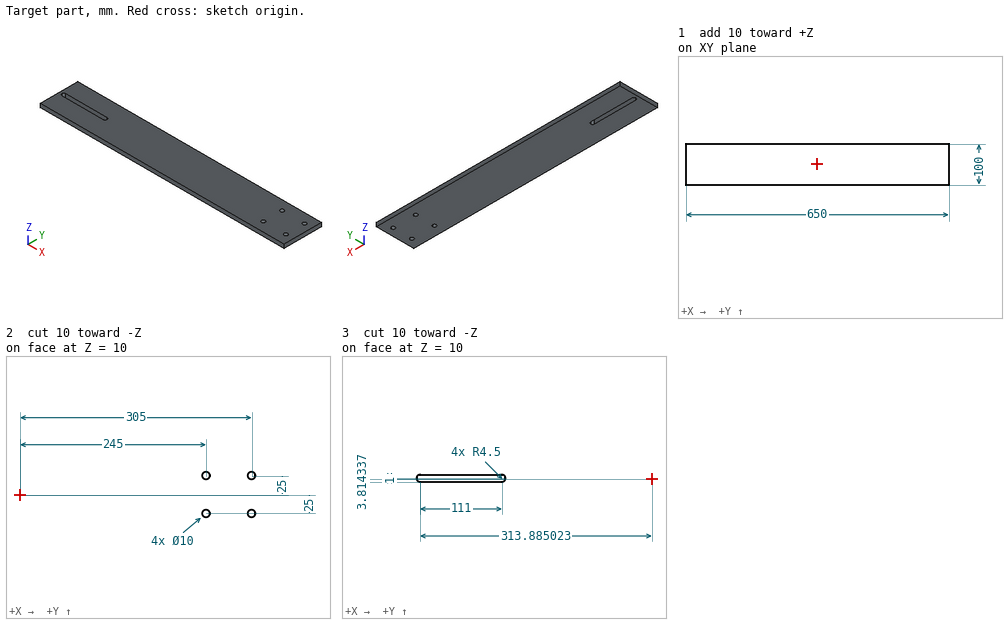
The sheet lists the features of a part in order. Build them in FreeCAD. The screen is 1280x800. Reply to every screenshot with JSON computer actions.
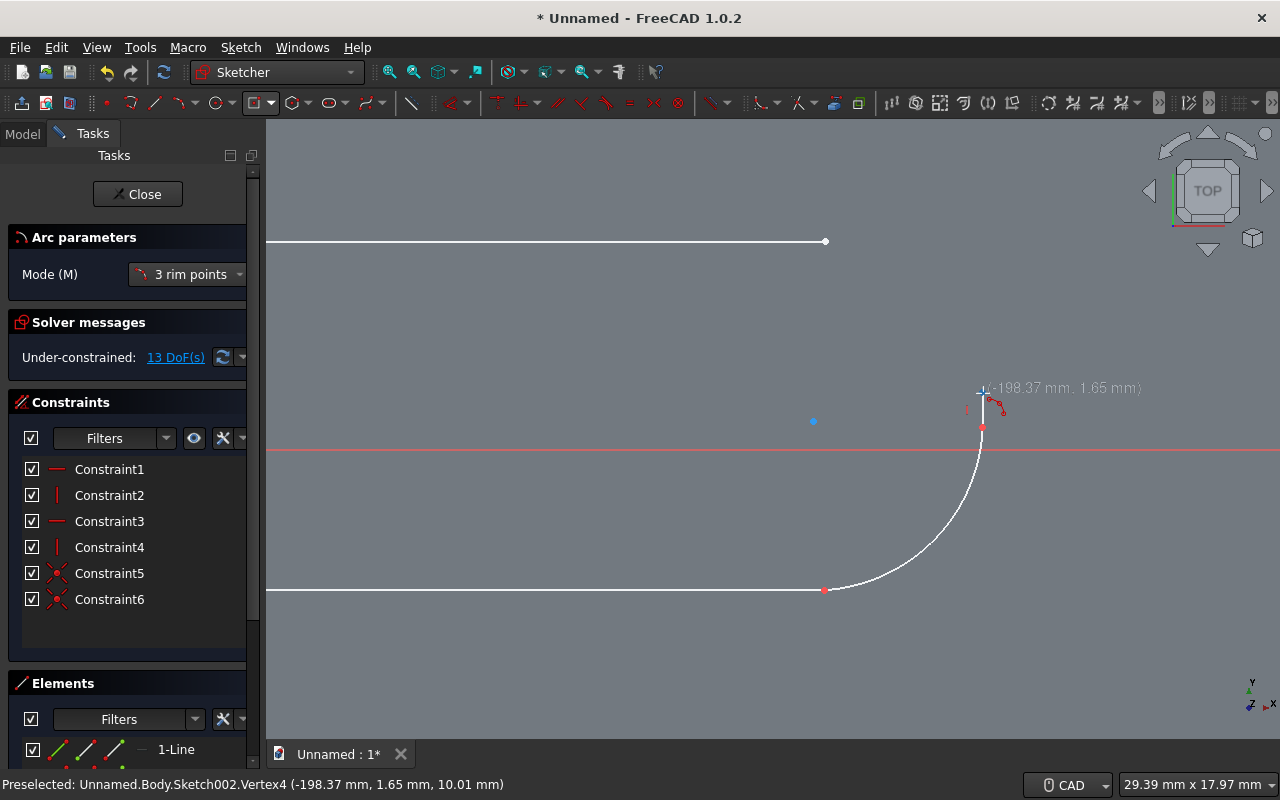
{"action": "scroll", "coordinate": [985, 432], "scroll_direction": "down", "scroll_amount": 10}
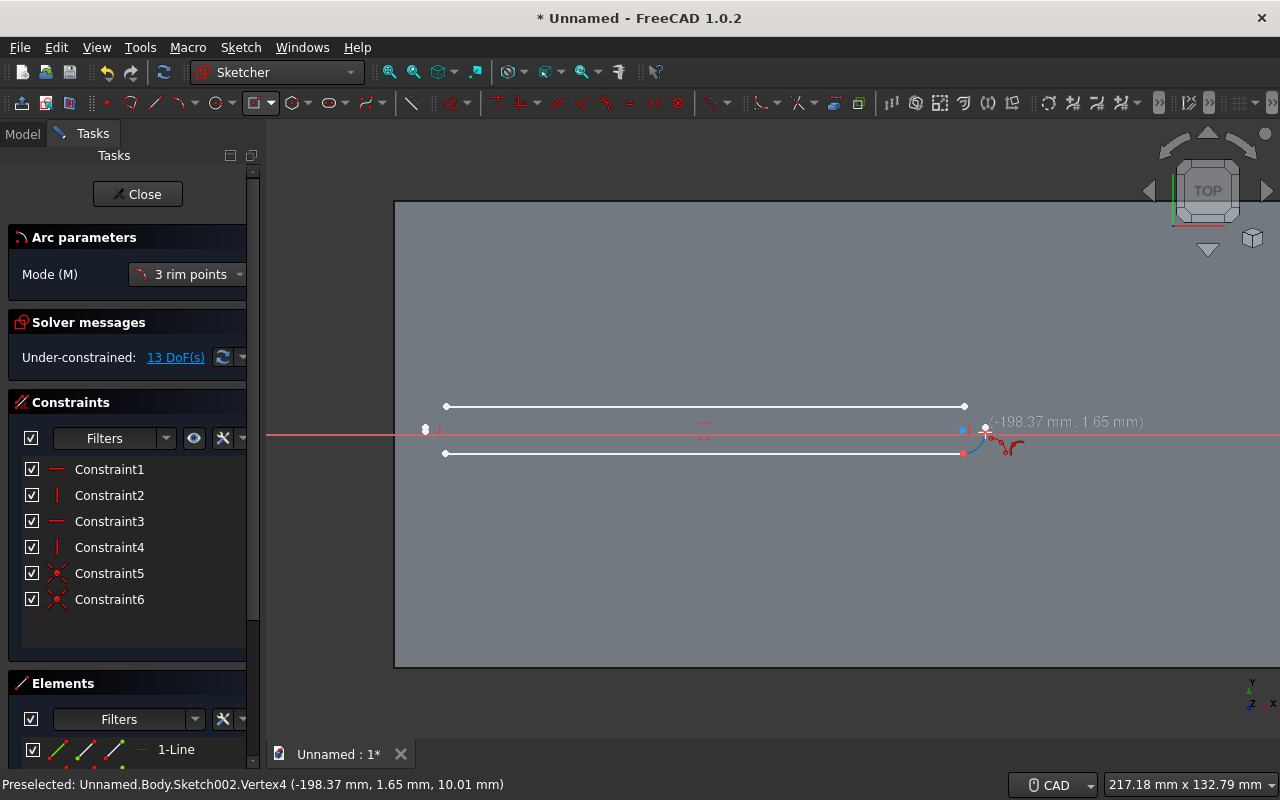
{"action": "left_click", "coordinate": [964, 407]}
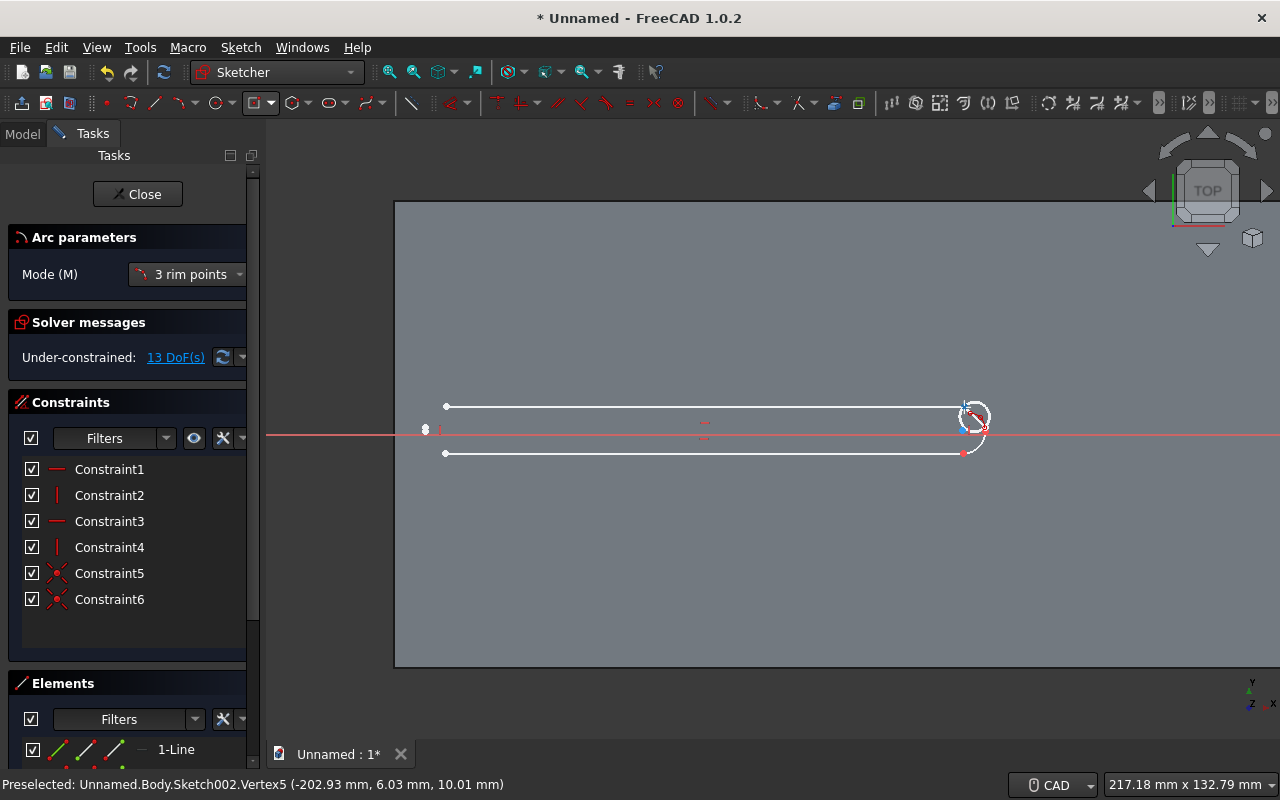
{"action": "scroll", "coordinate": [979, 412], "scroll_direction": "up", "scroll_amount": 5}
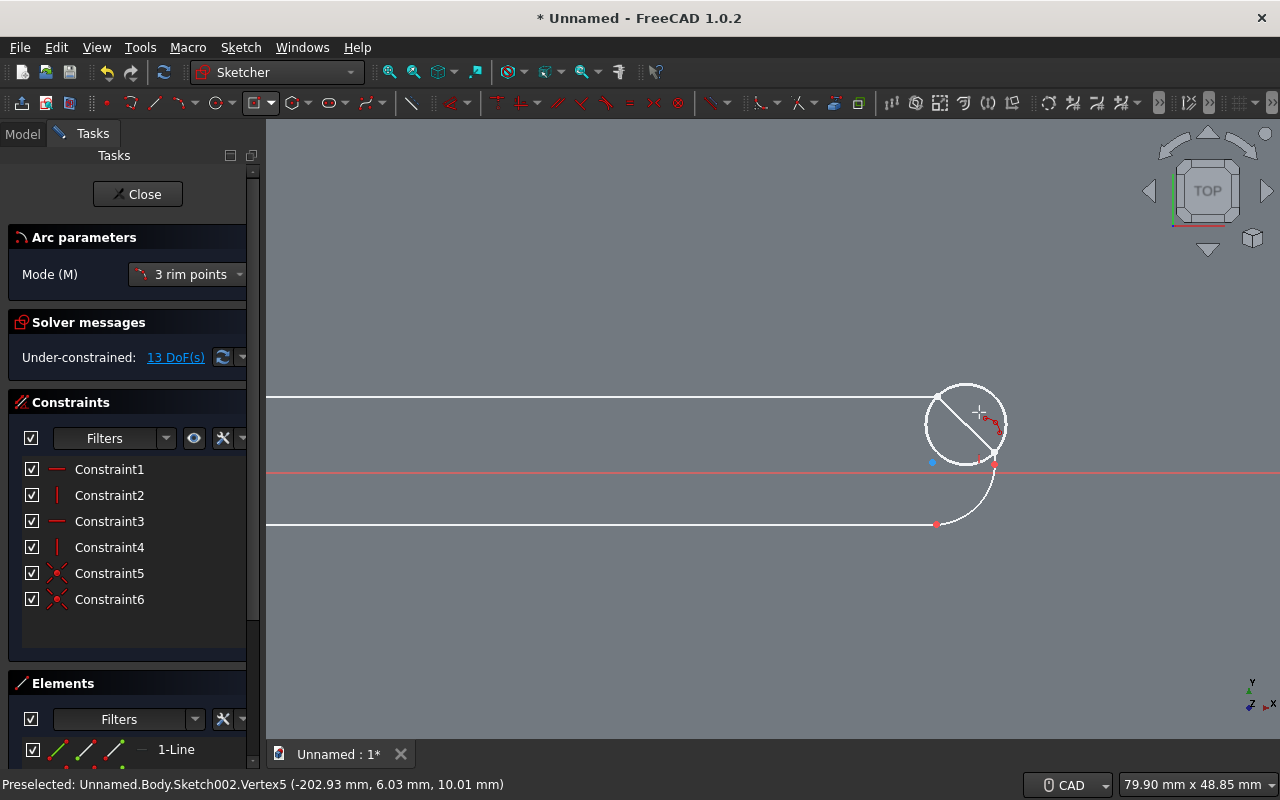
{"action": "left_click", "coordinate": [978, 411]}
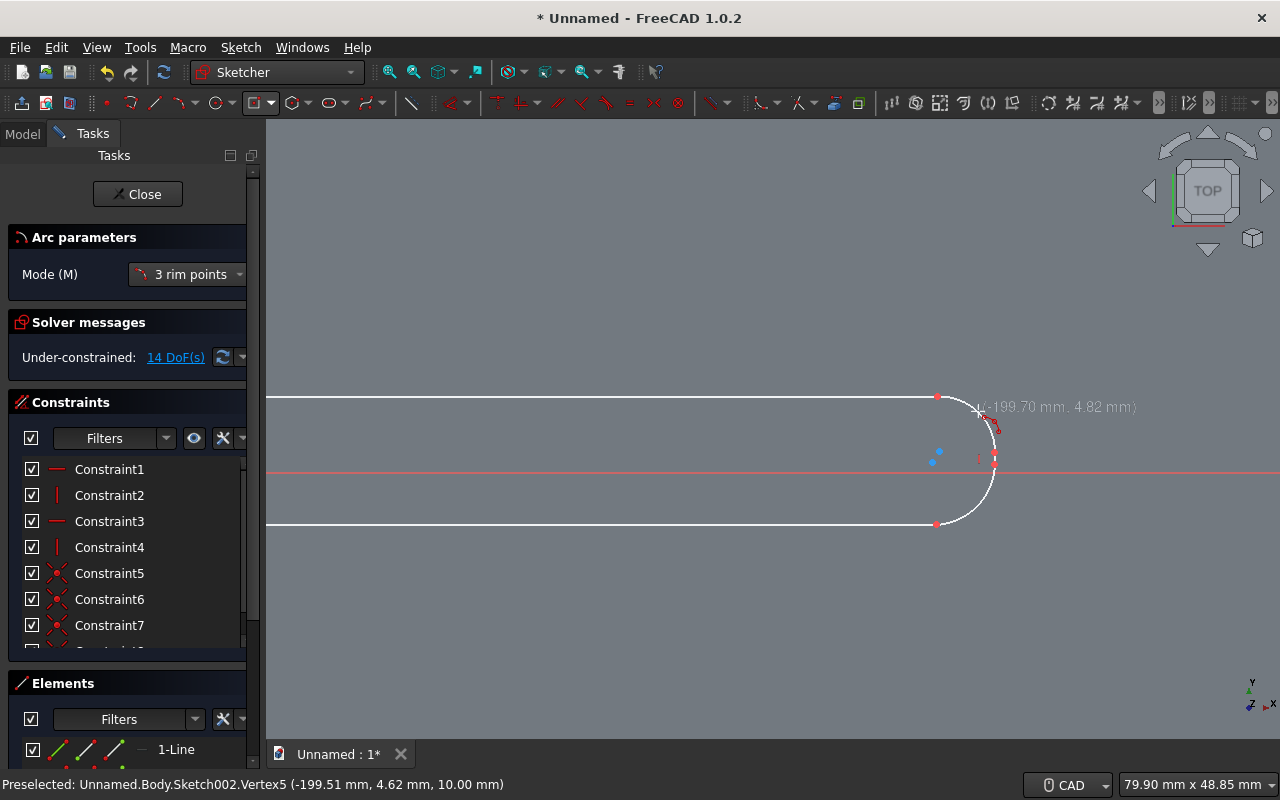
{"action": "scroll", "coordinate": [979, 412], "scroll_direction": "down", "scroll_amount": 5}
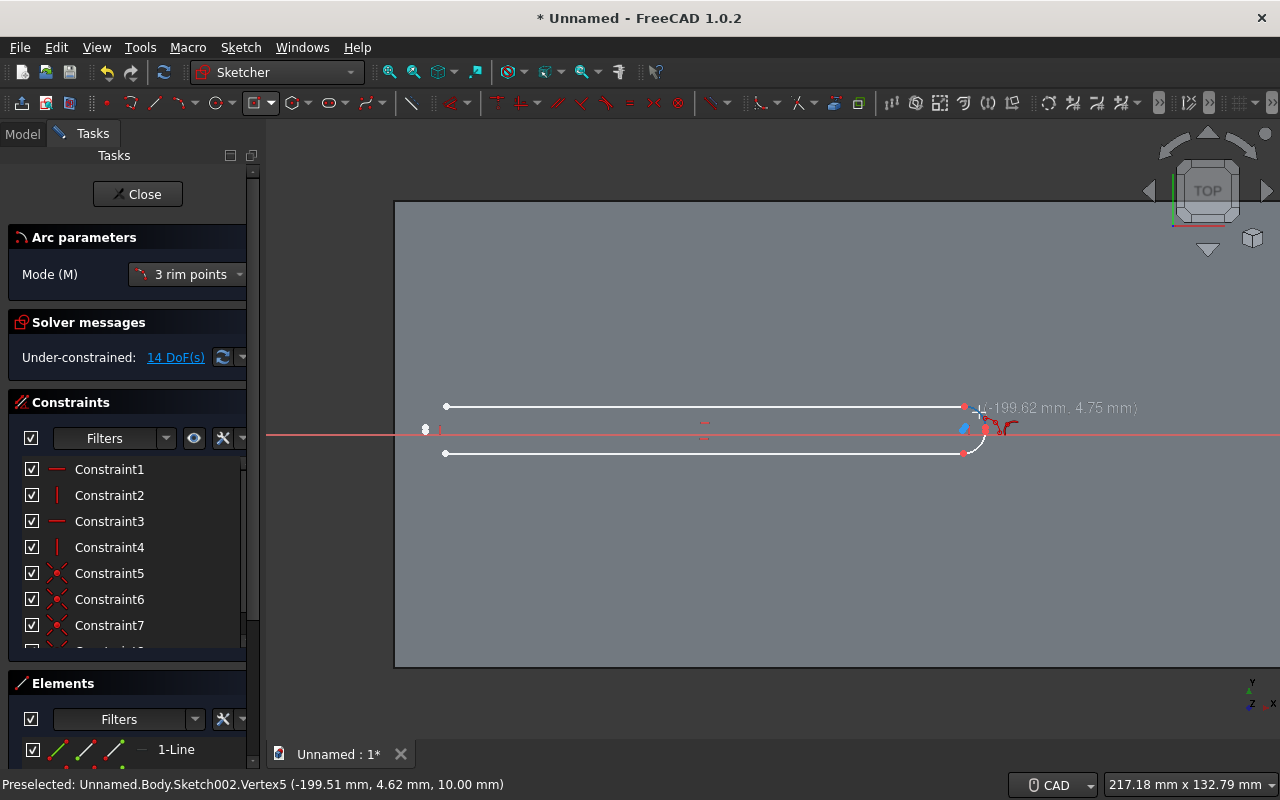
{"action": "left_click", "coordinate": [446, 407]}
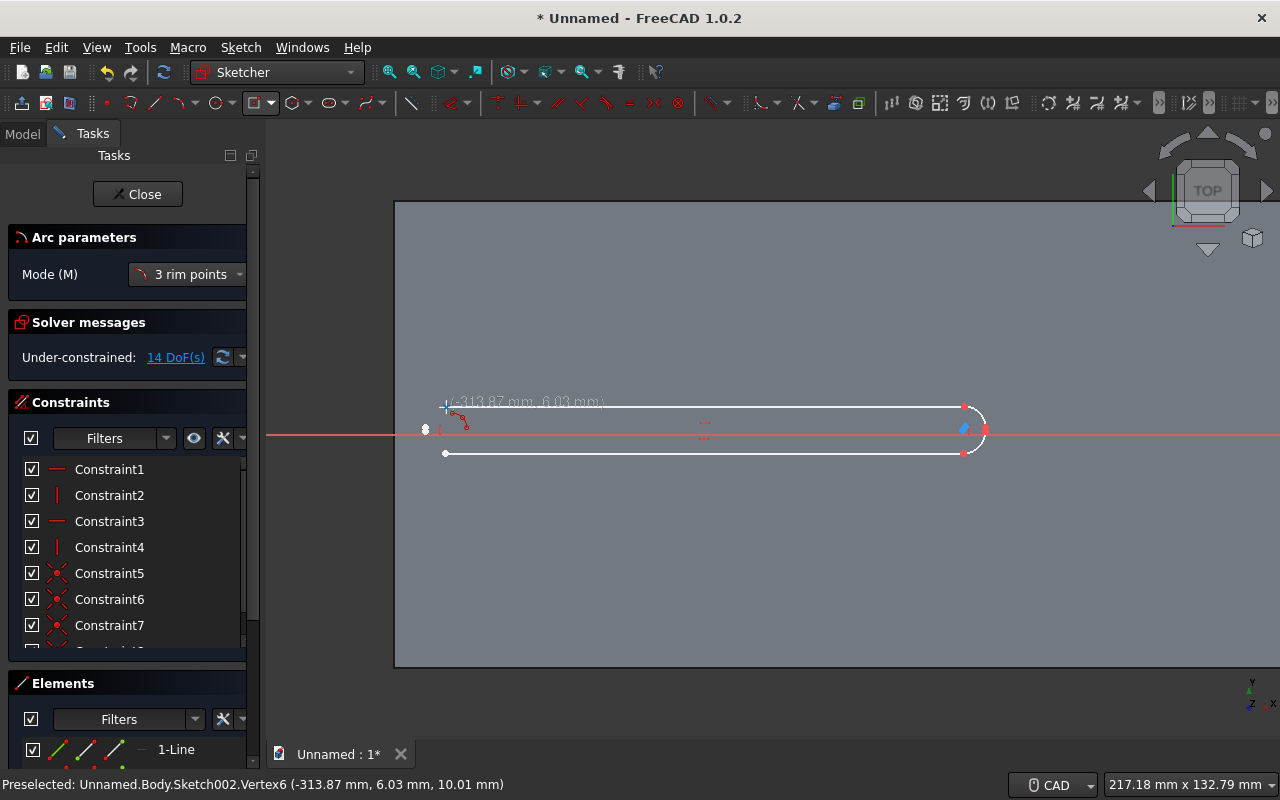
{"action": "scroll", "coordinate": [425, 427], "scroll_direction": "up", "scroll_amount": 10}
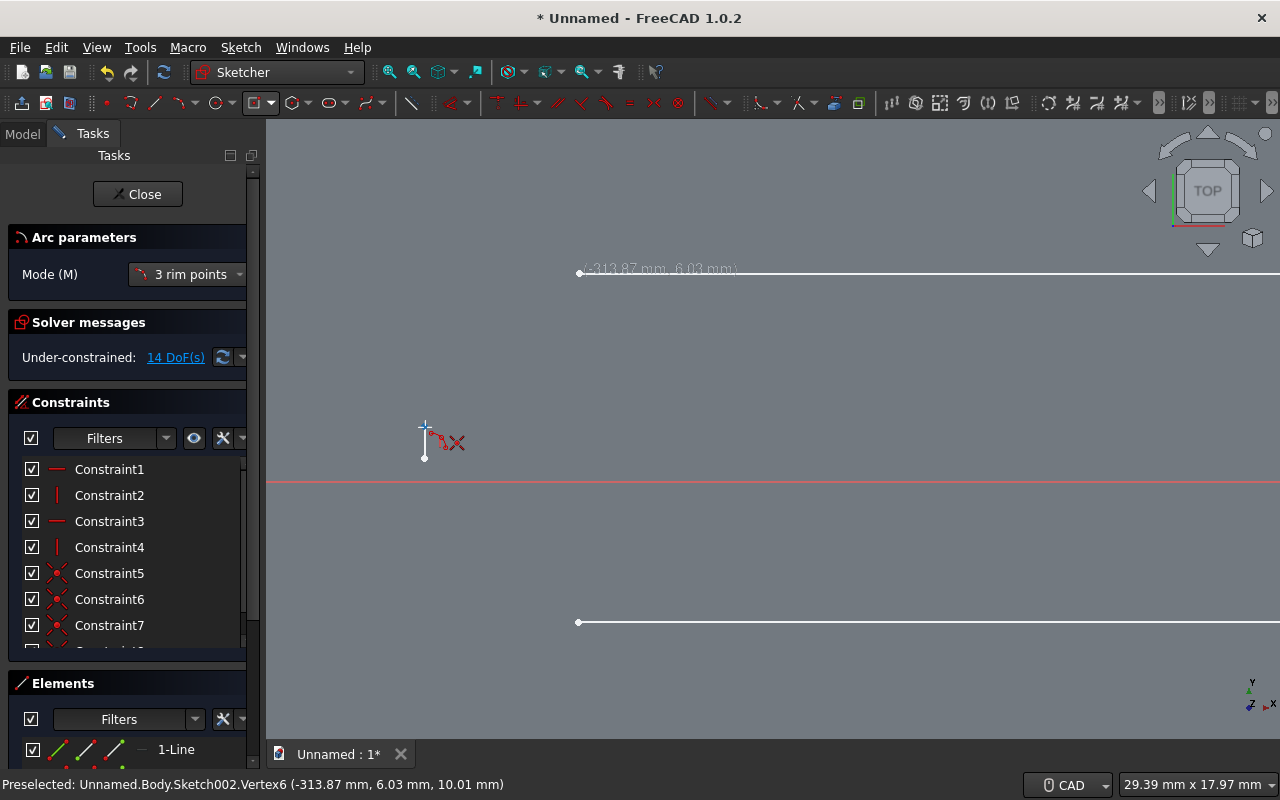
{"action": "left_click", "coordinate": [425, 427]}
{"action": "left_click", "coordinate": [469, 314]}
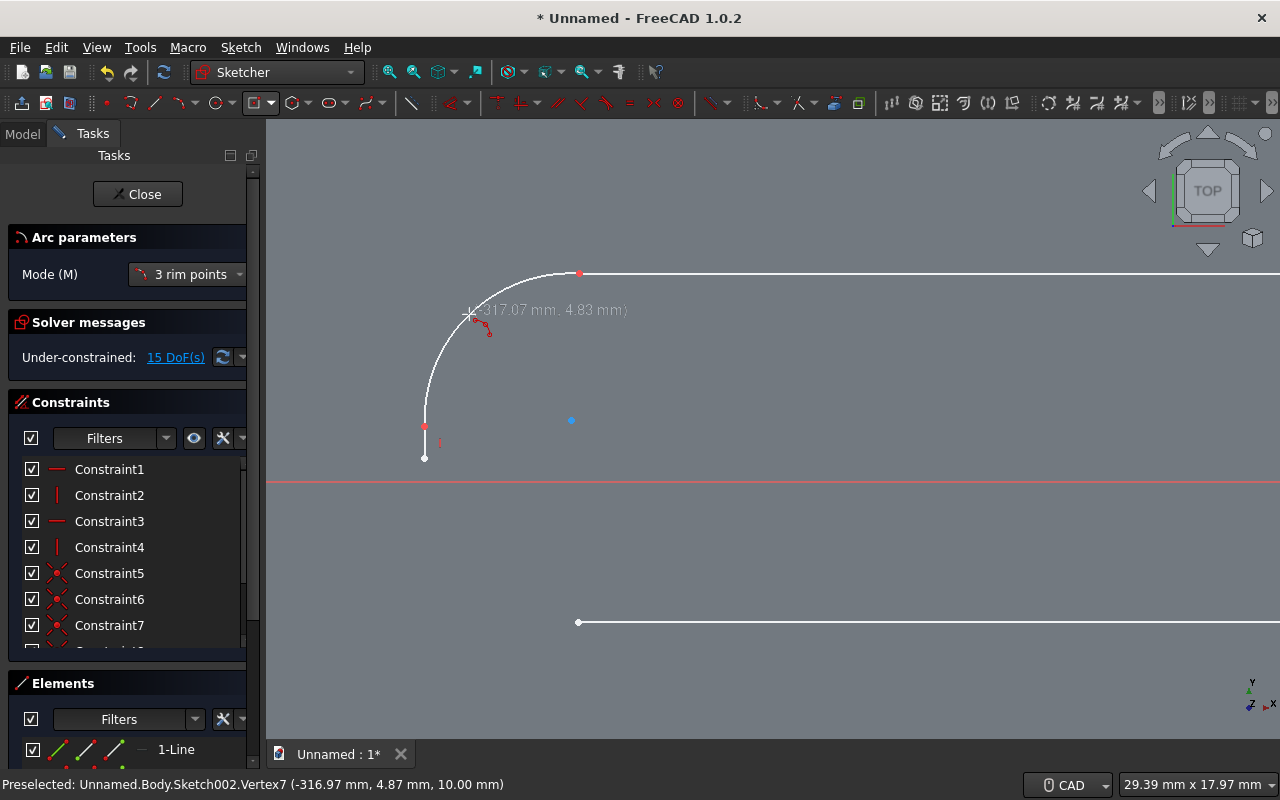
{"action": "left_click", "coordinate": [425, 459]}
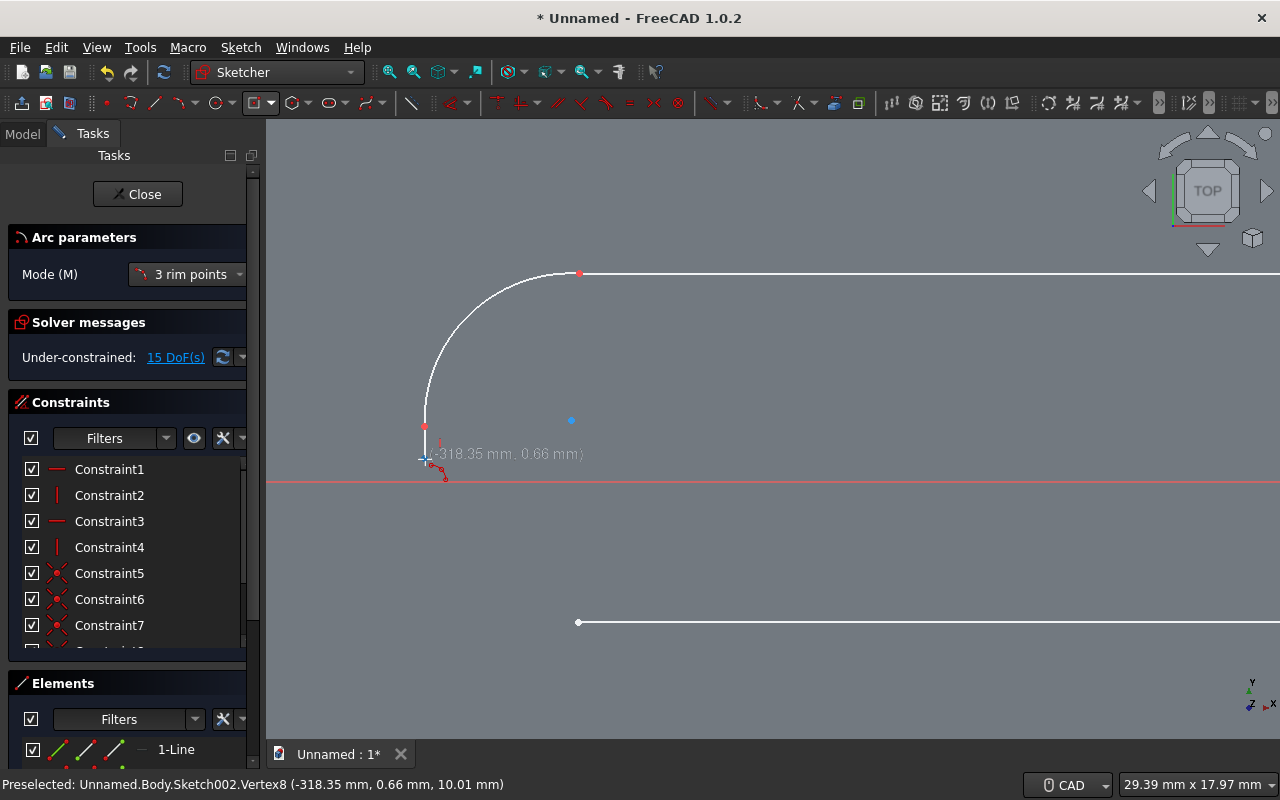
{"action": "scroll", "coordinate": [424, 427], "scroll_direction": "down", "scroll_amount": 10}